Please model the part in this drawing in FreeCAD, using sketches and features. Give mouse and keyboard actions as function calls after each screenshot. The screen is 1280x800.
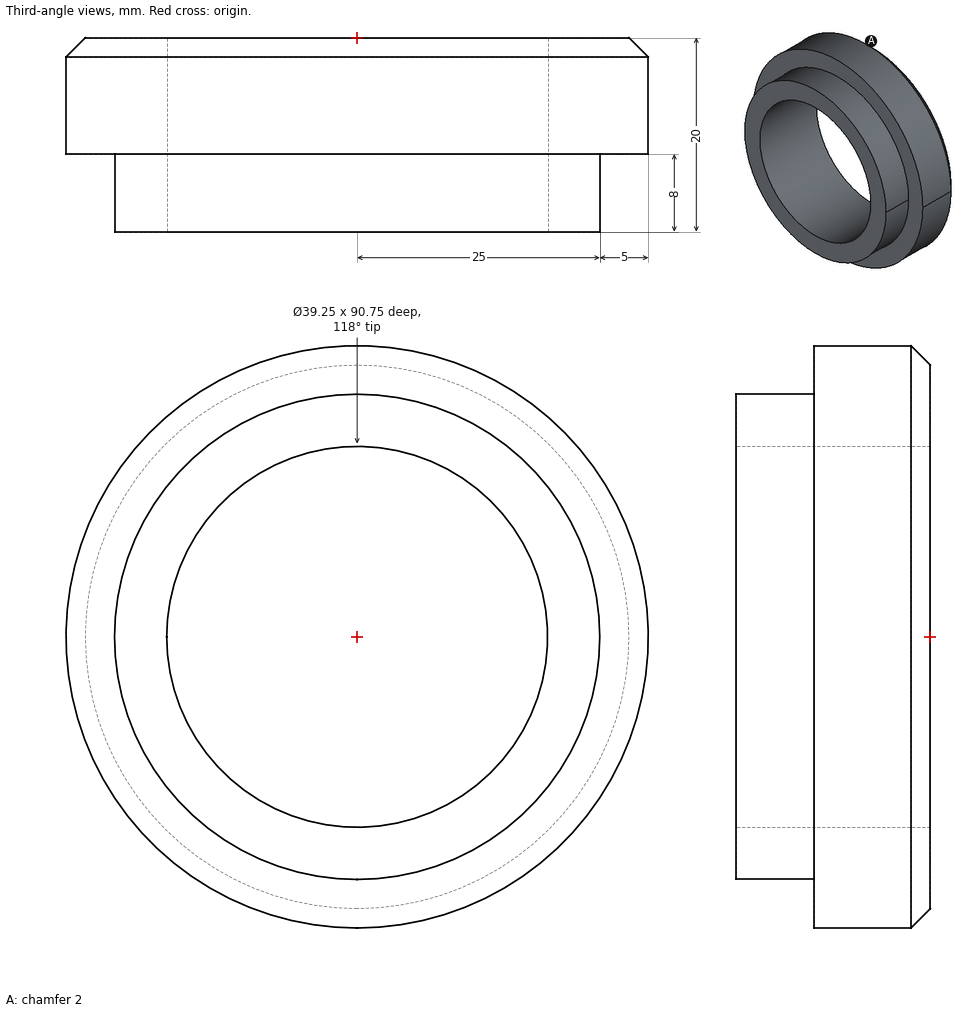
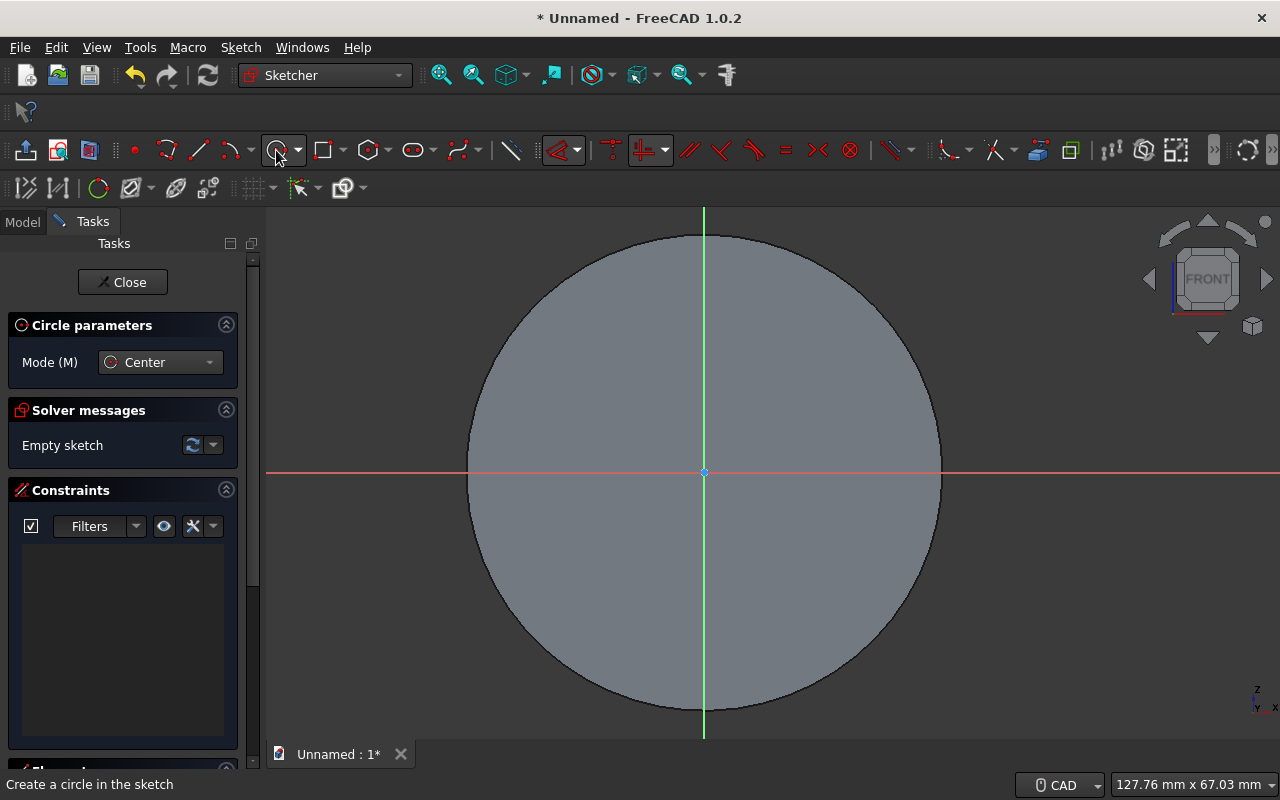
click(704, 473)
move(814, 363)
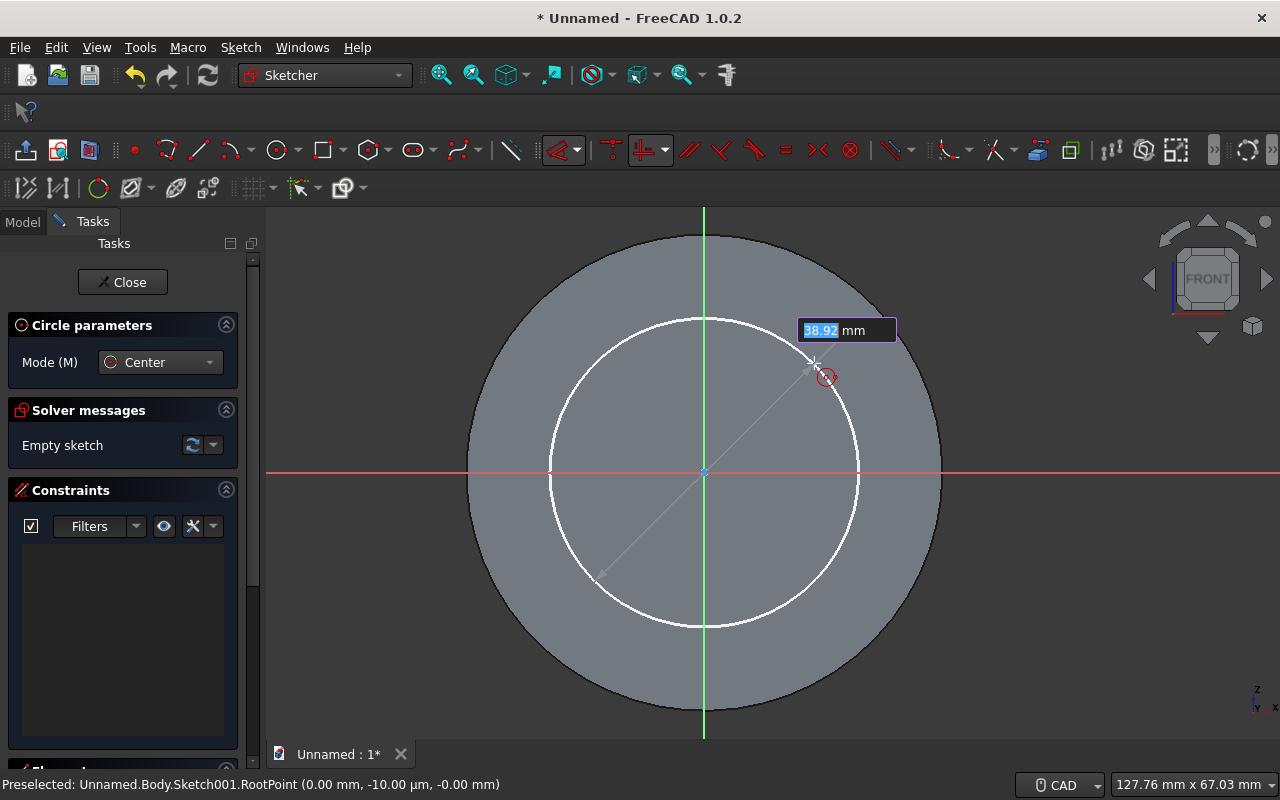
text(39.25)
key(Return)
key(Escape)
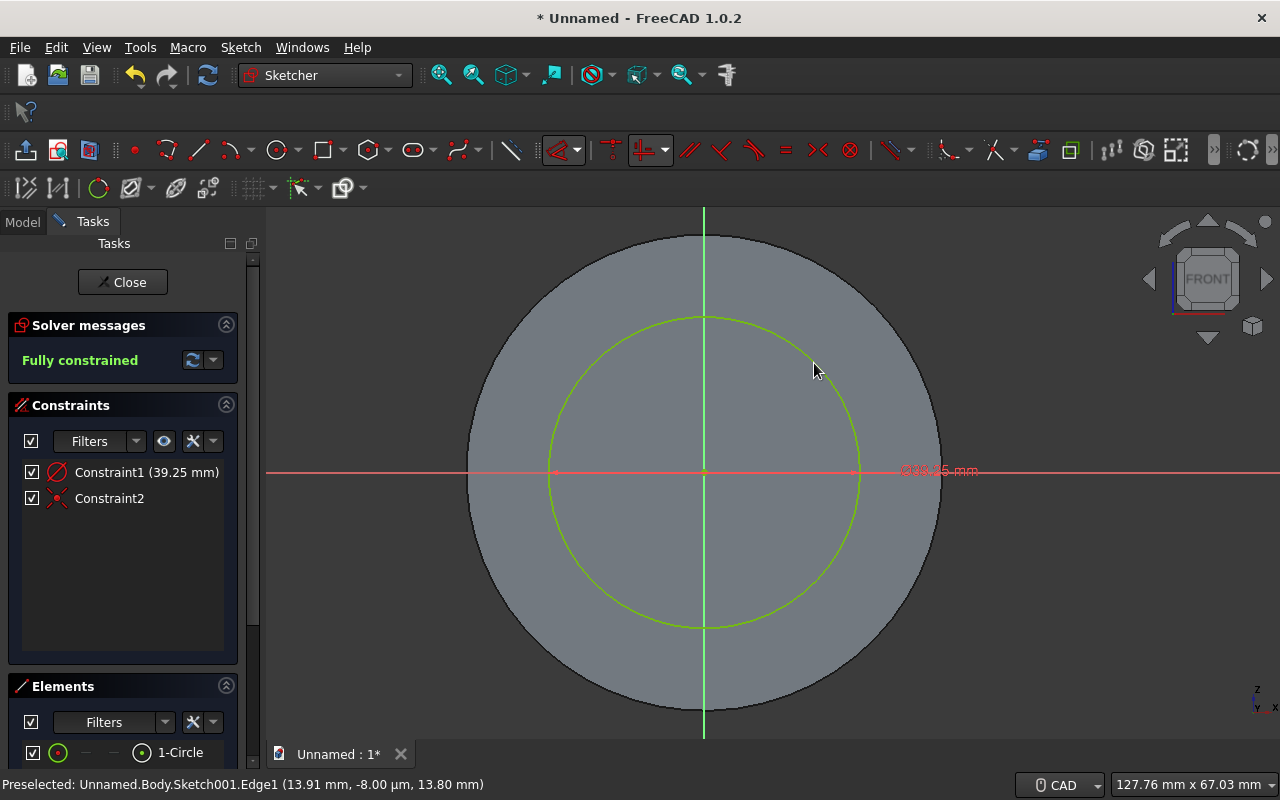
click(123, 282)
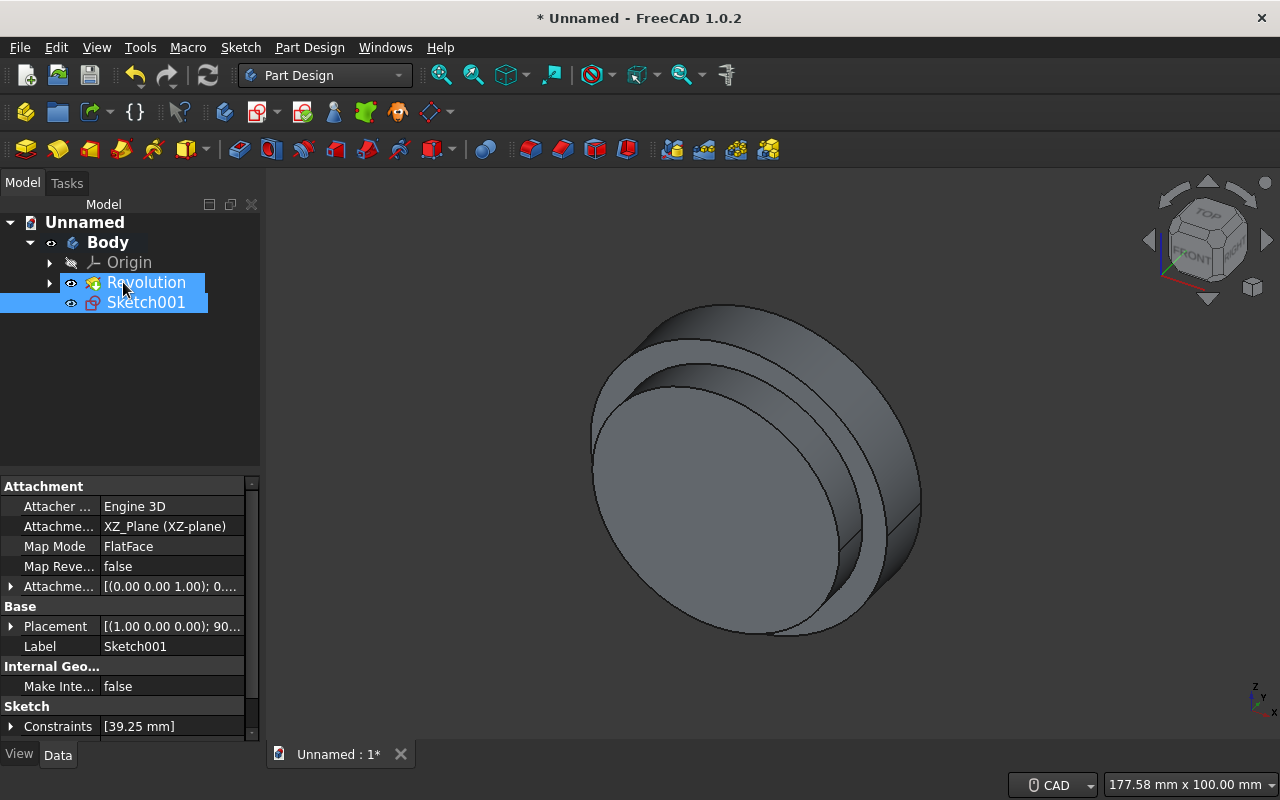
click(272, 150)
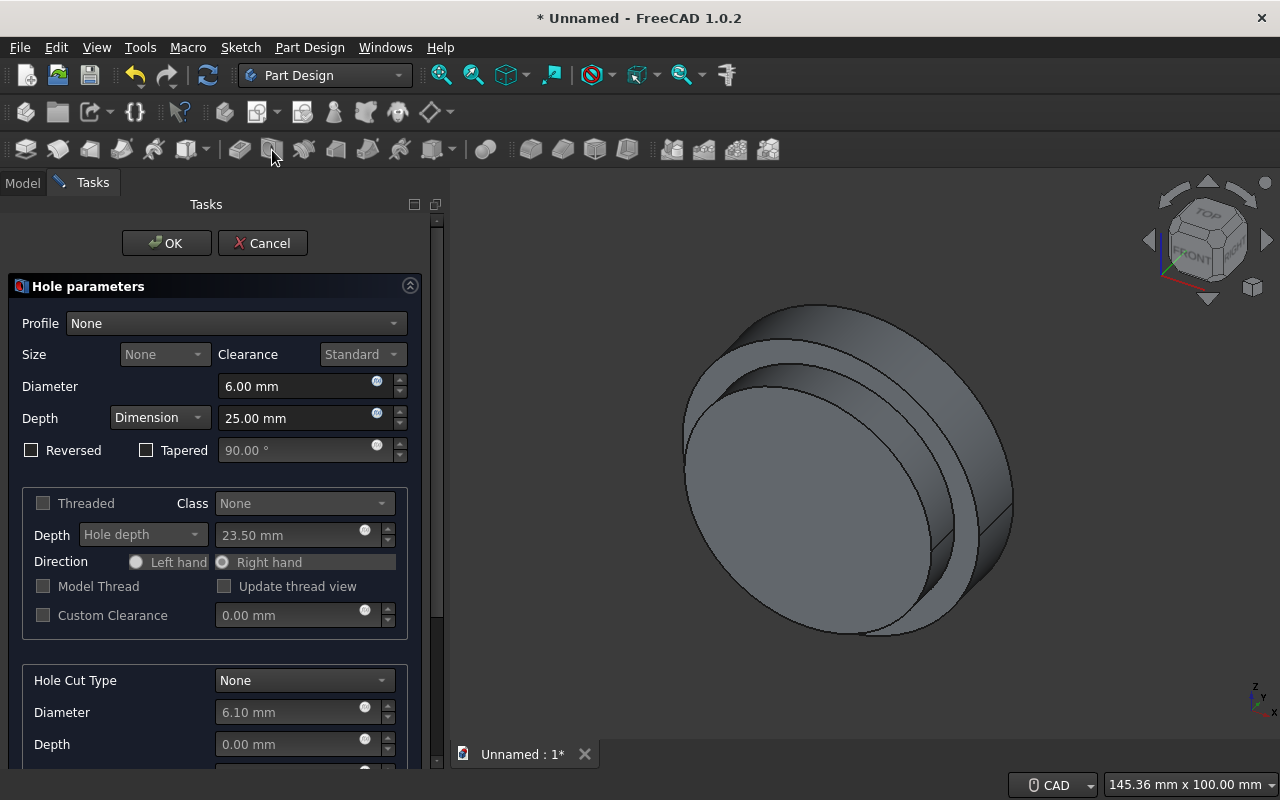
triple_click(305, 386)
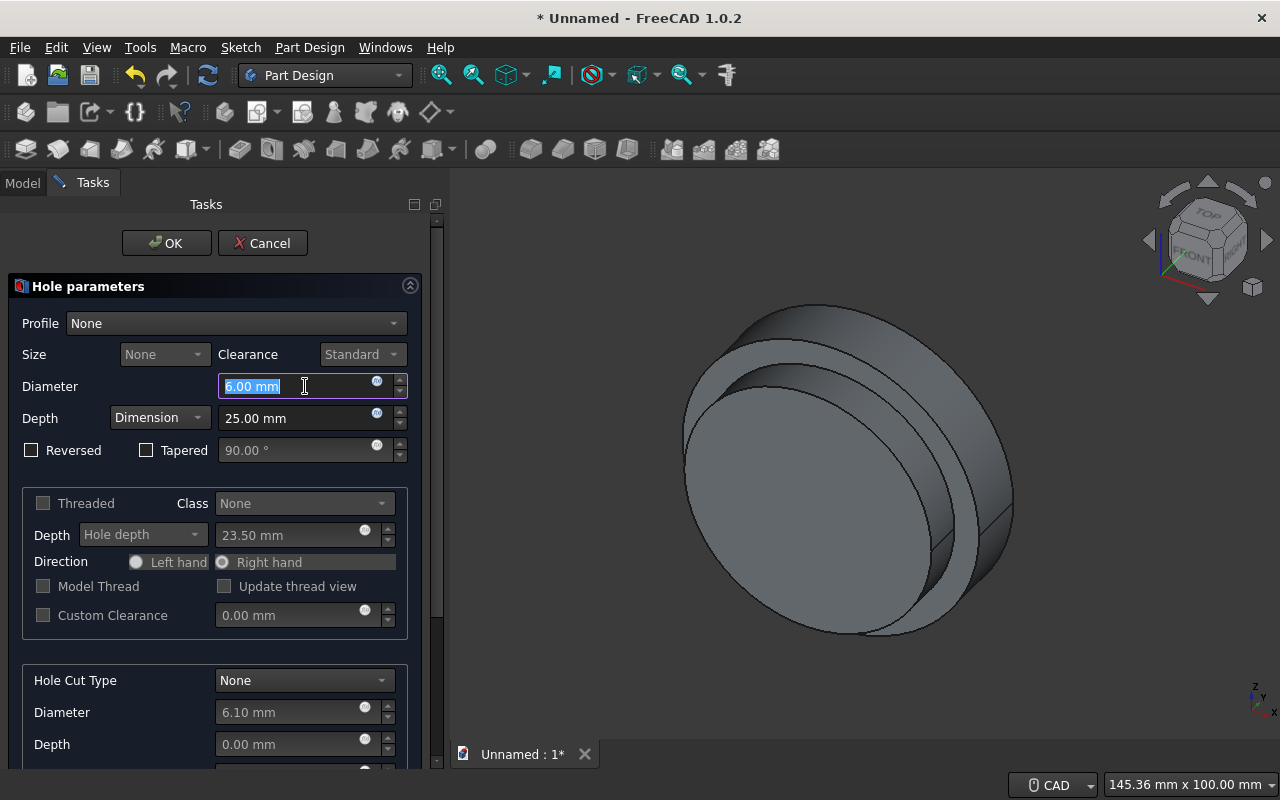
text(39.25)
key(Tab)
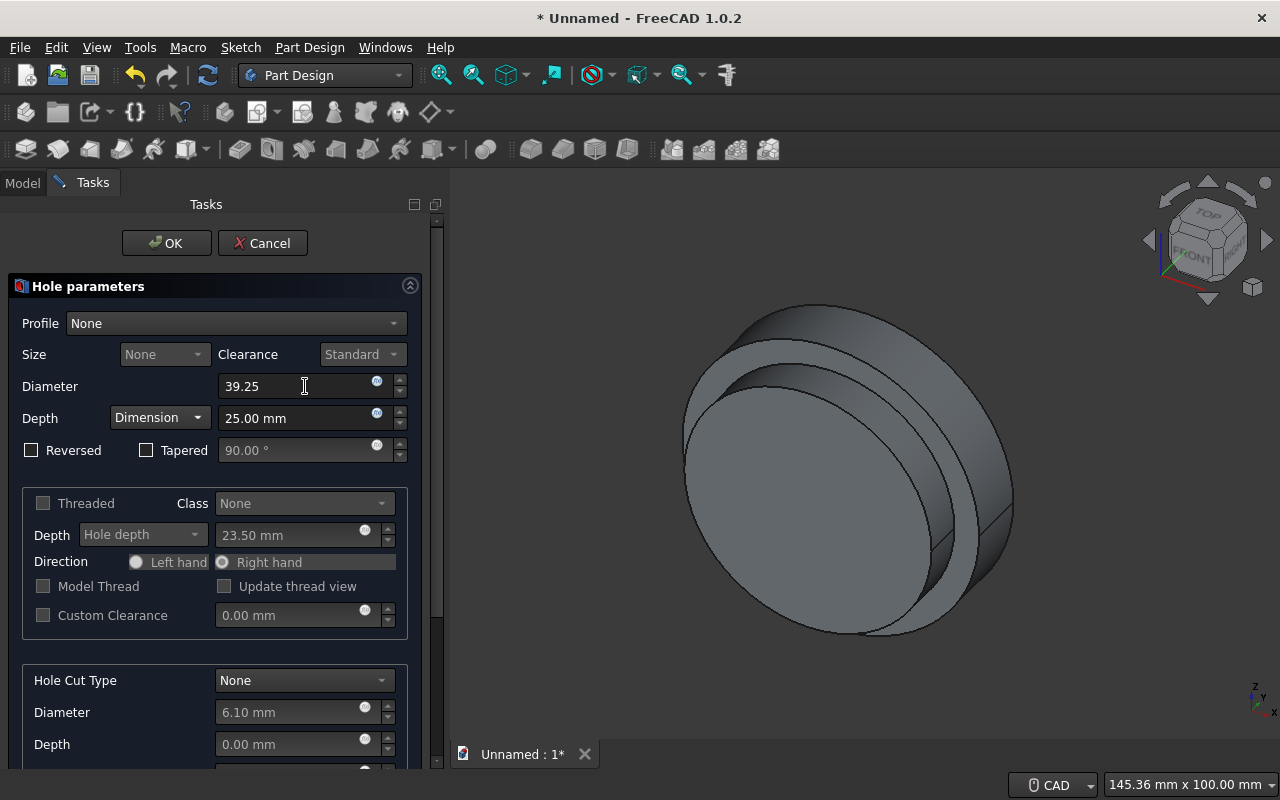
triple_click(305, 418)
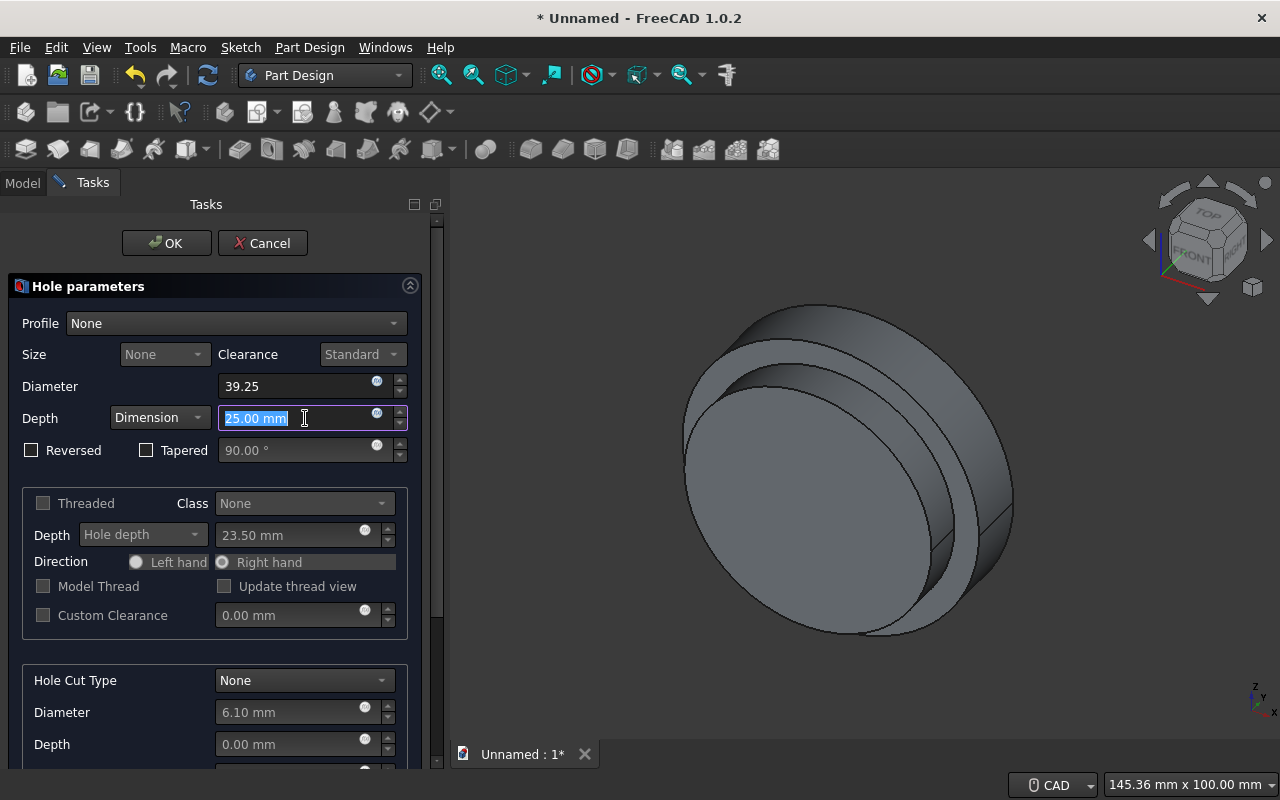
text(90.75)
key(Tab)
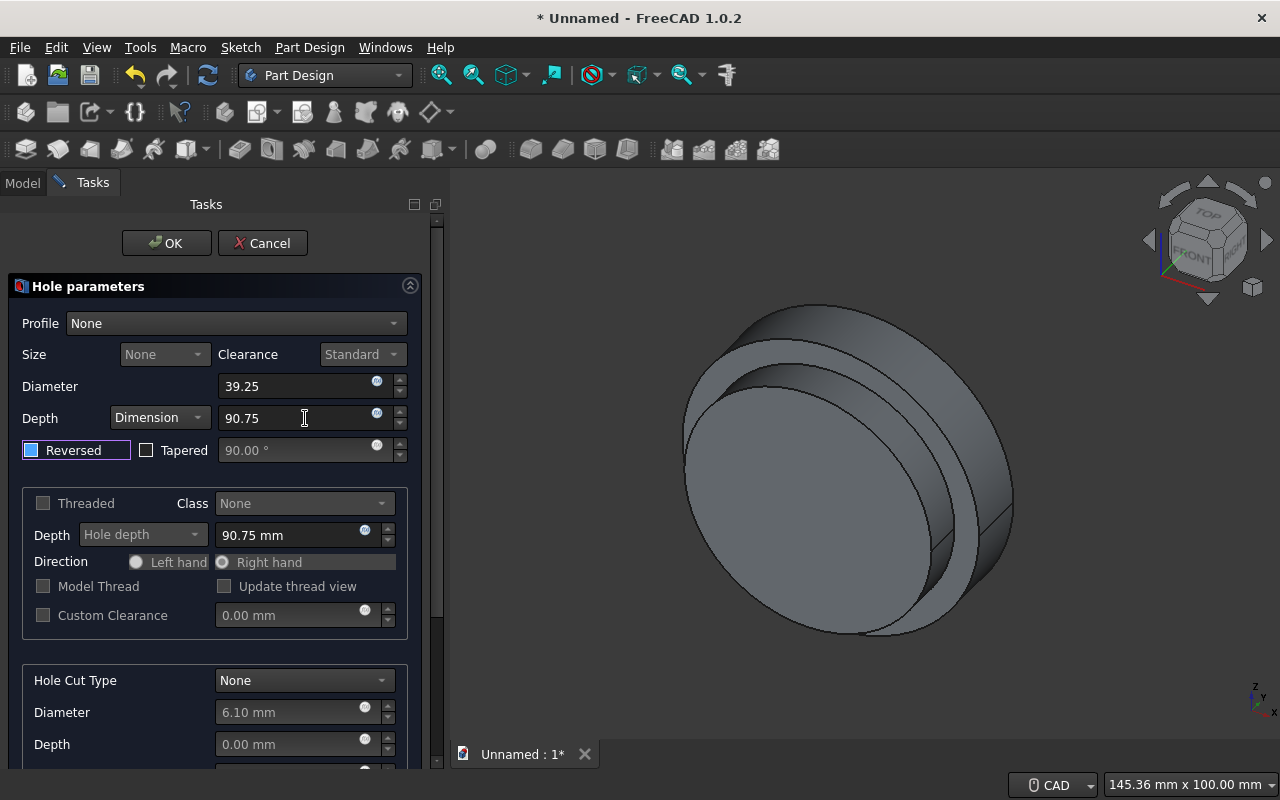
click(30, 450)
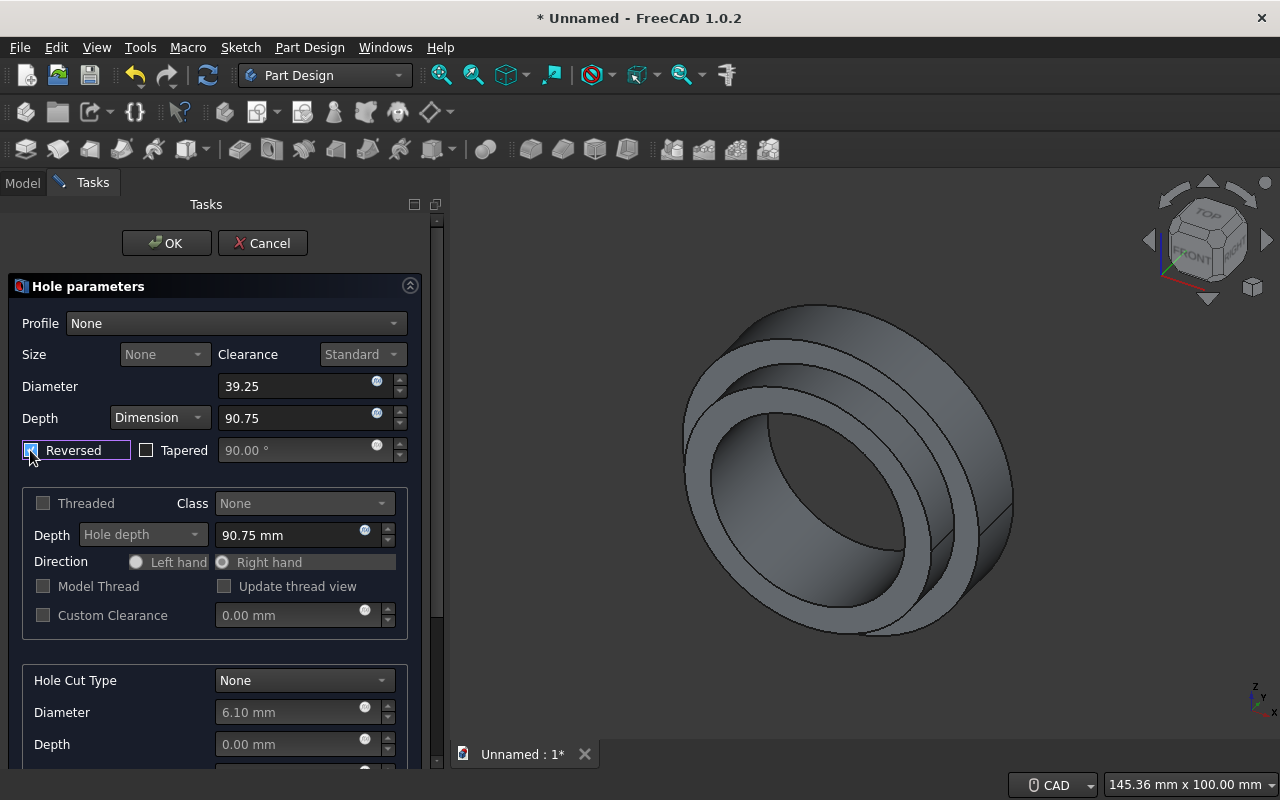
click(167, 243)